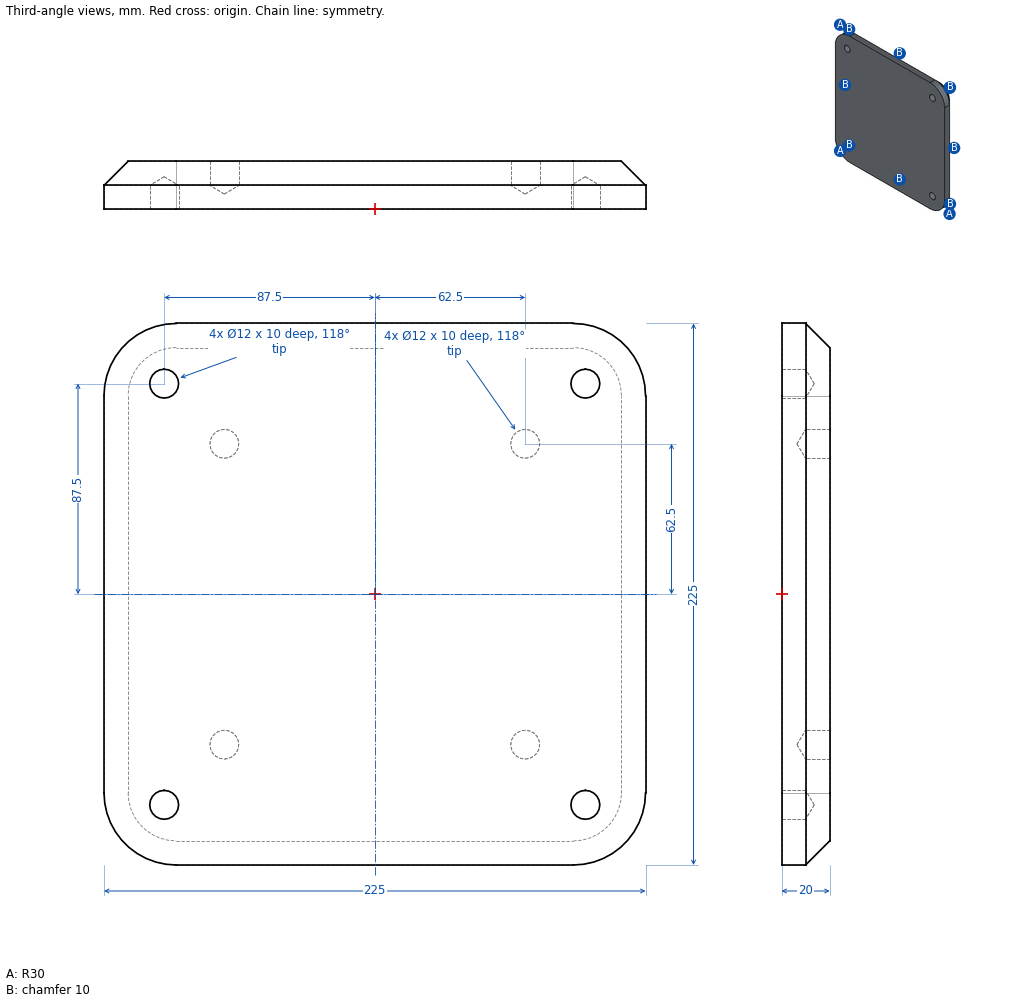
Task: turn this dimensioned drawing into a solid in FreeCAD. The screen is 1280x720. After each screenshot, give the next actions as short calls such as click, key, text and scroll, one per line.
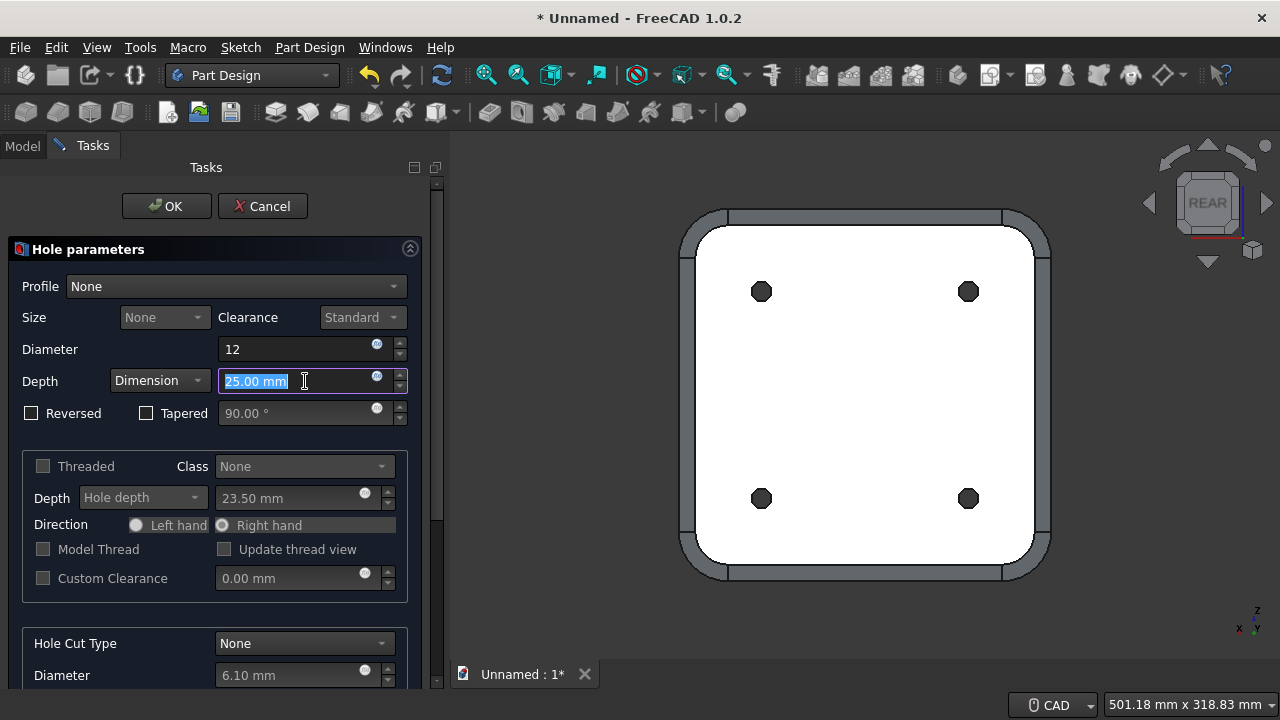
text(10)
key(Tab)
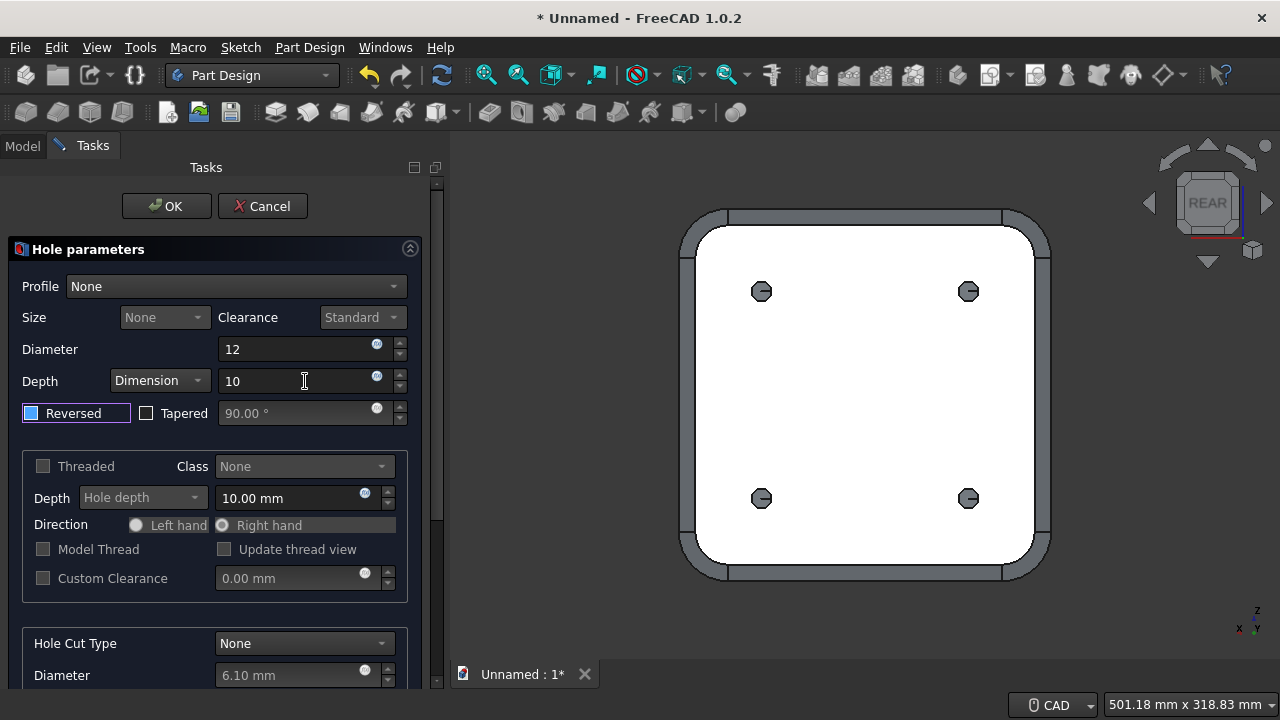
click(167, 206)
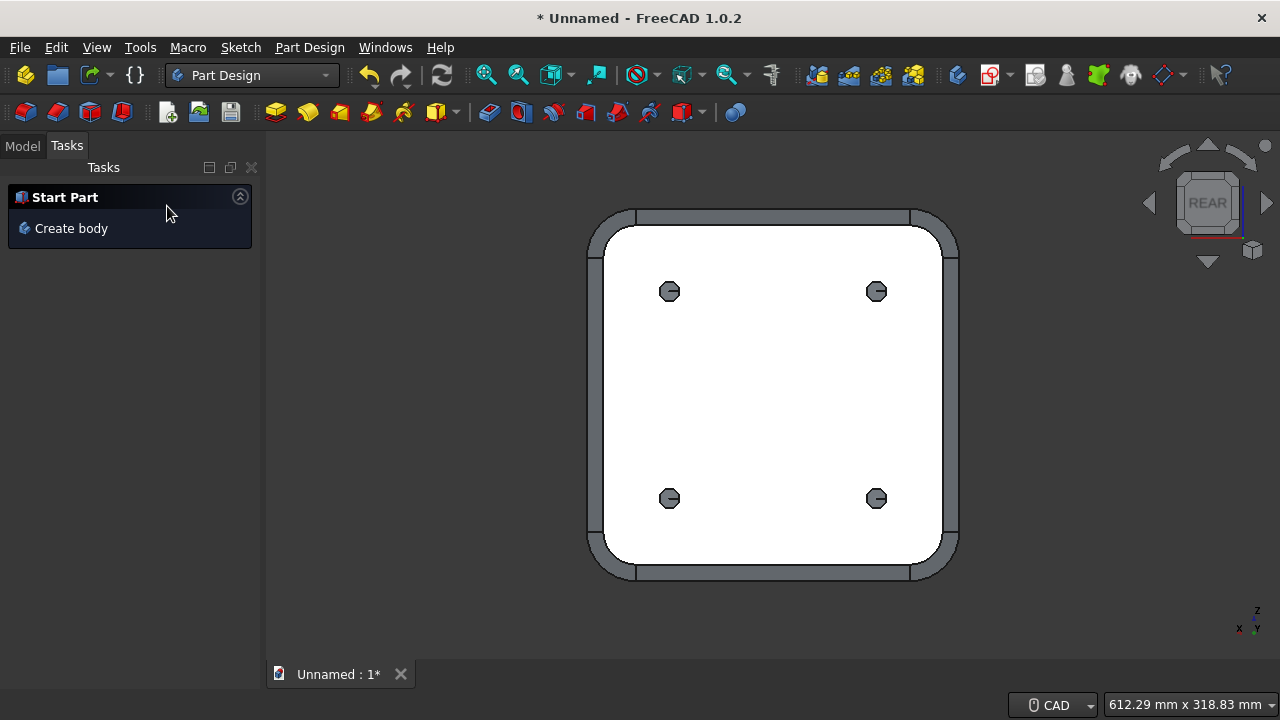
key(0)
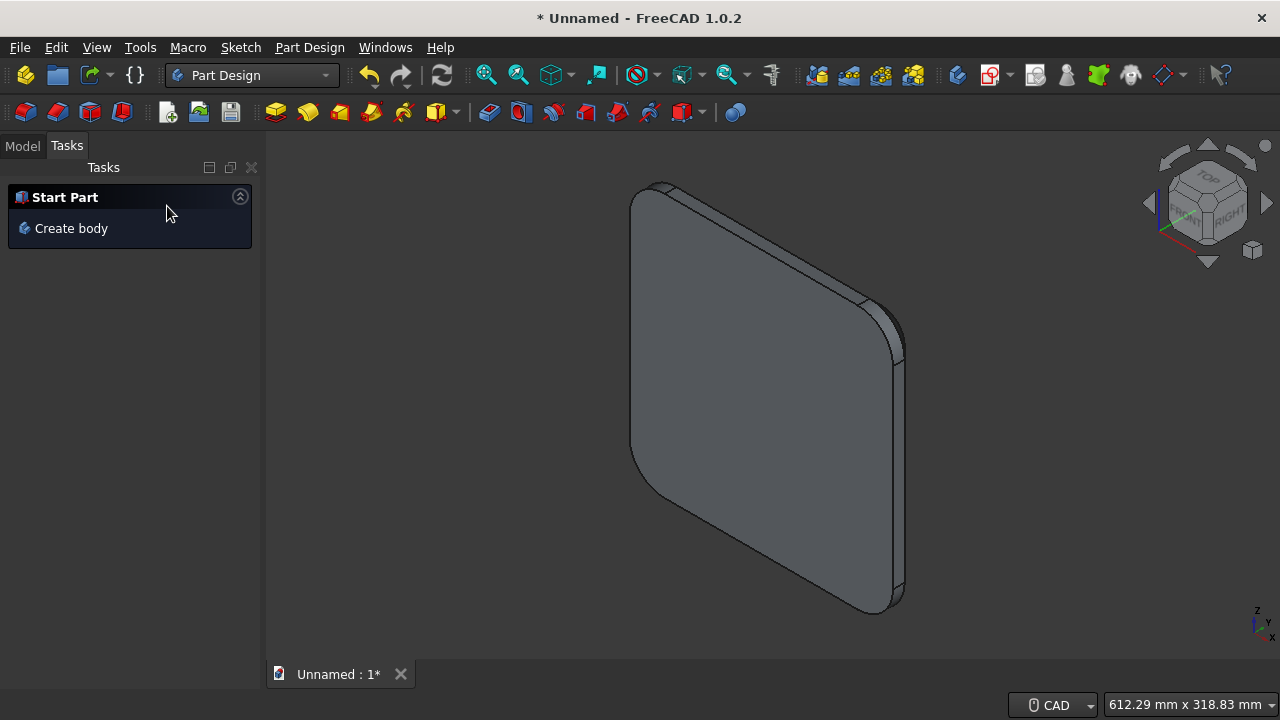
click(761, 401)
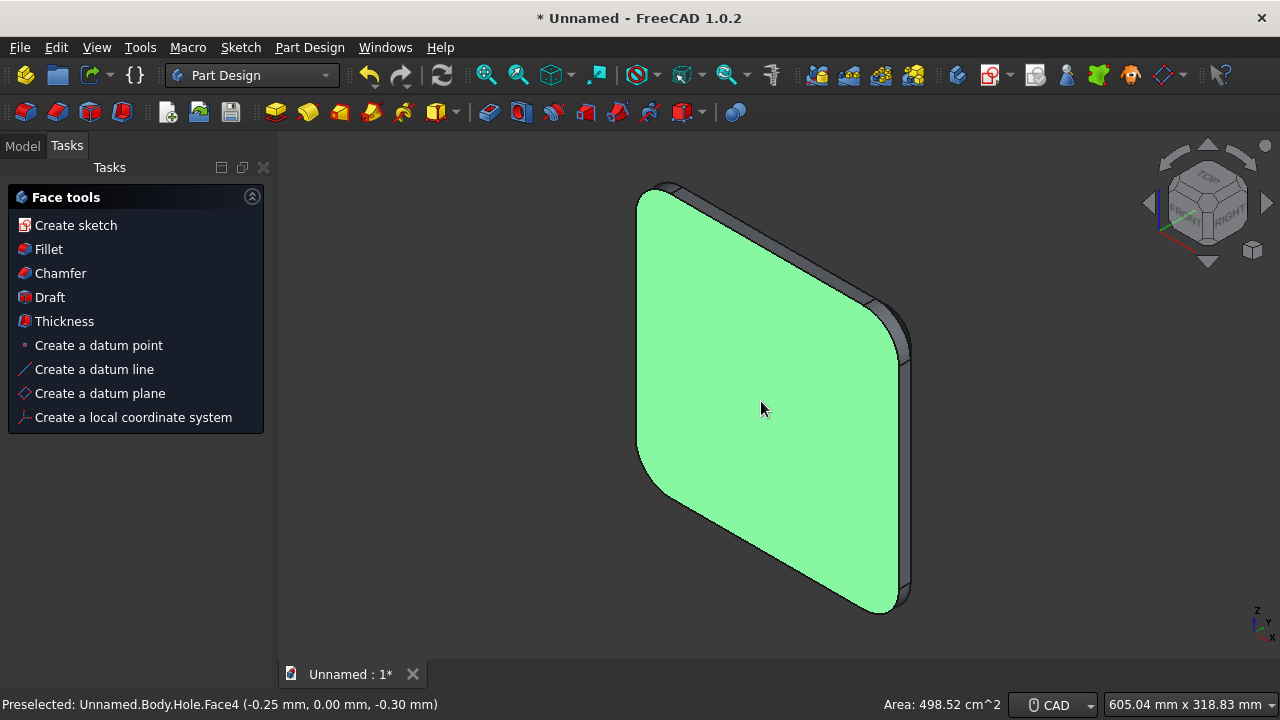
click(990, 76)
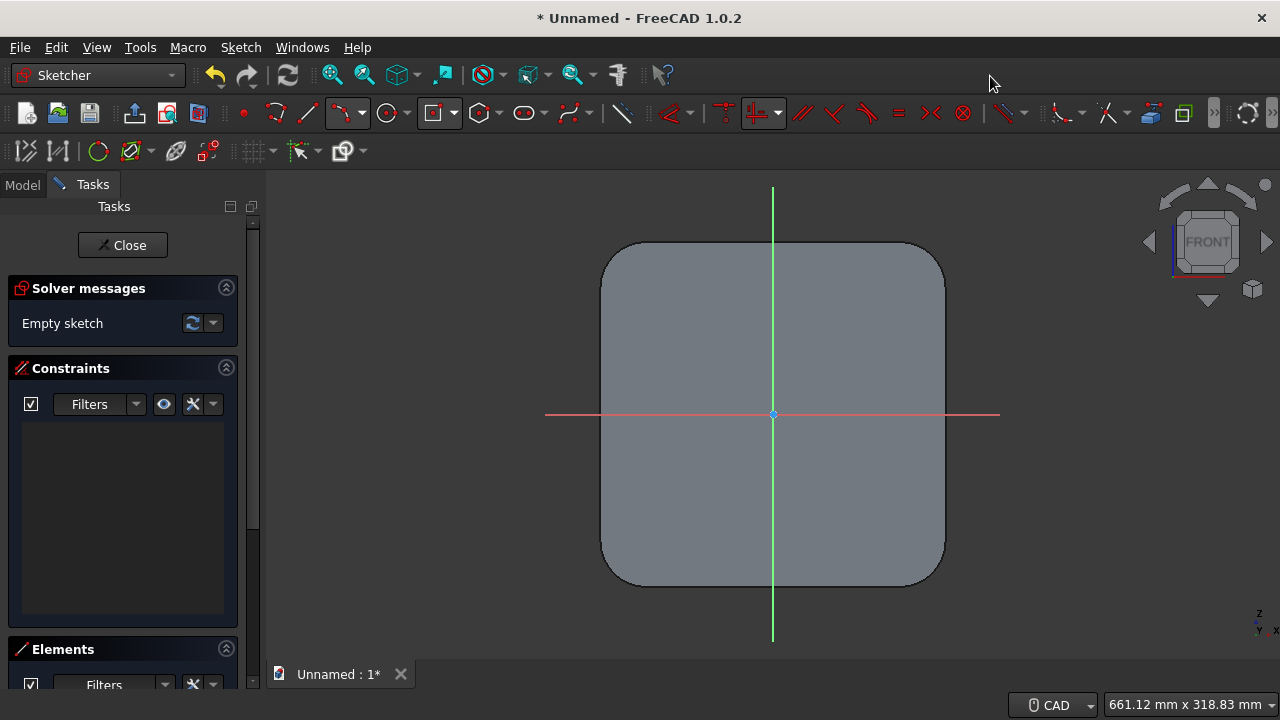
click(388, 114)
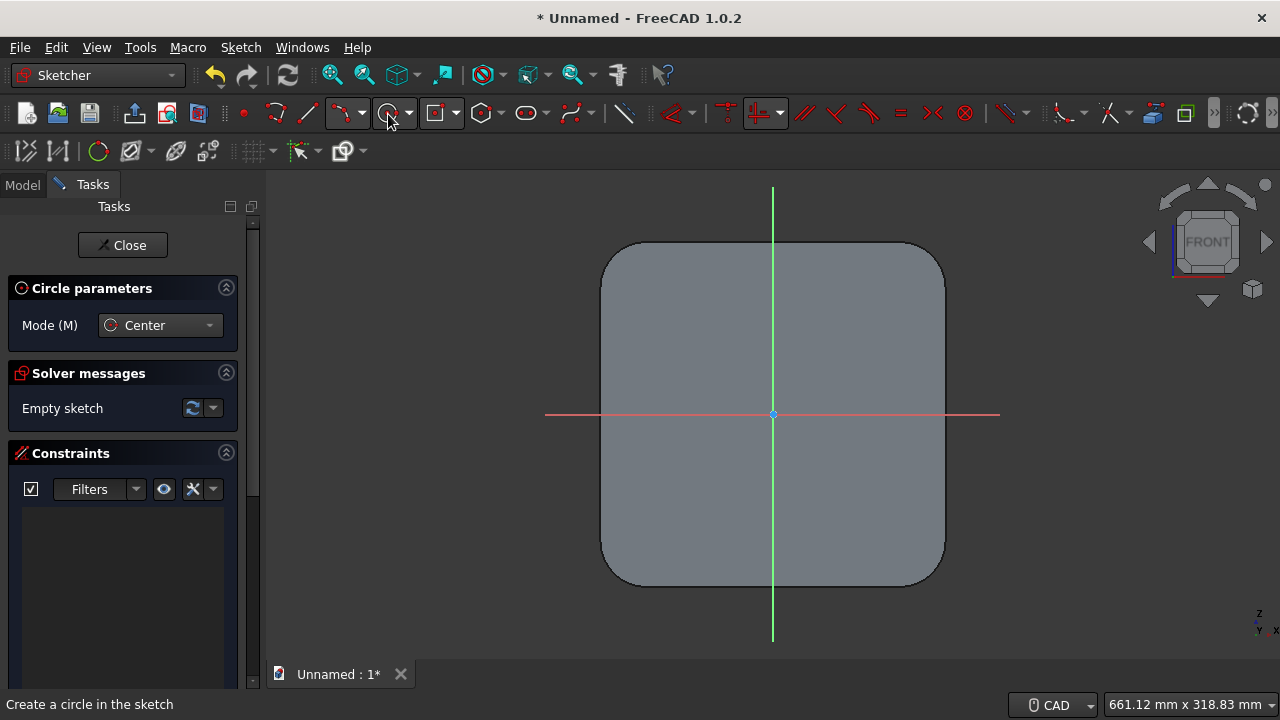
scroll(639, 280, up, 5)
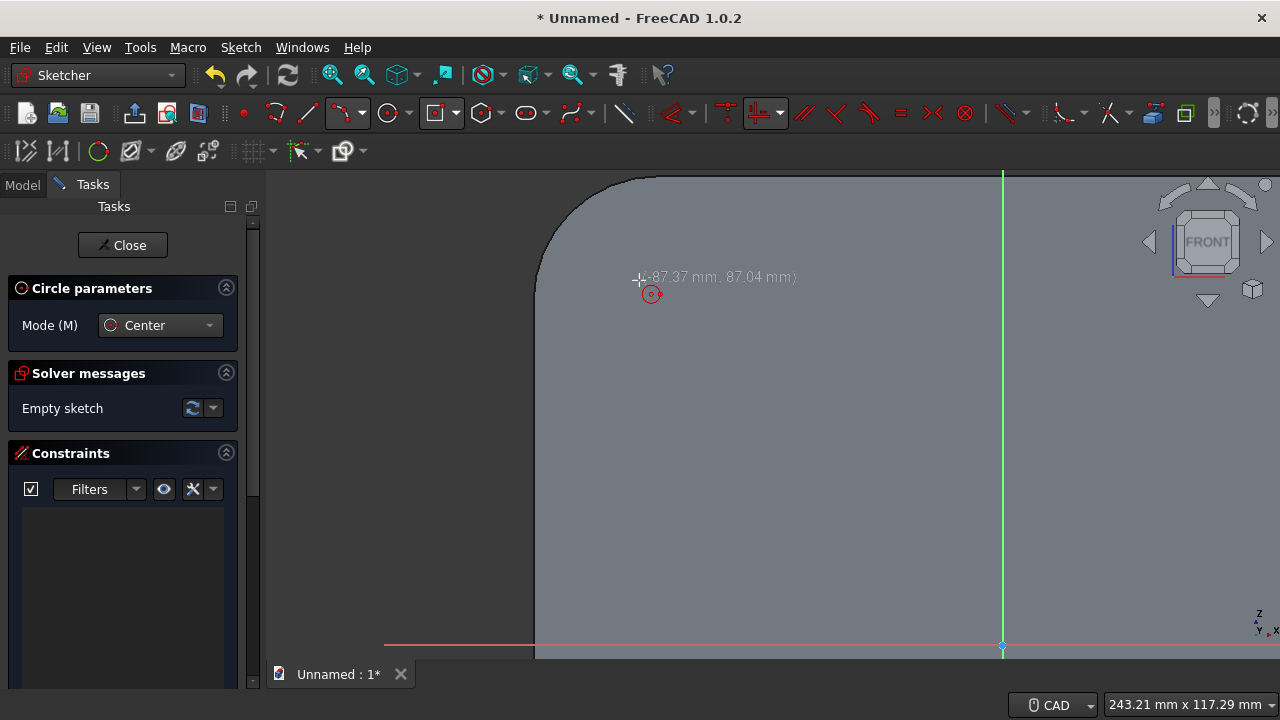
click(638, 280)
click(656, 263)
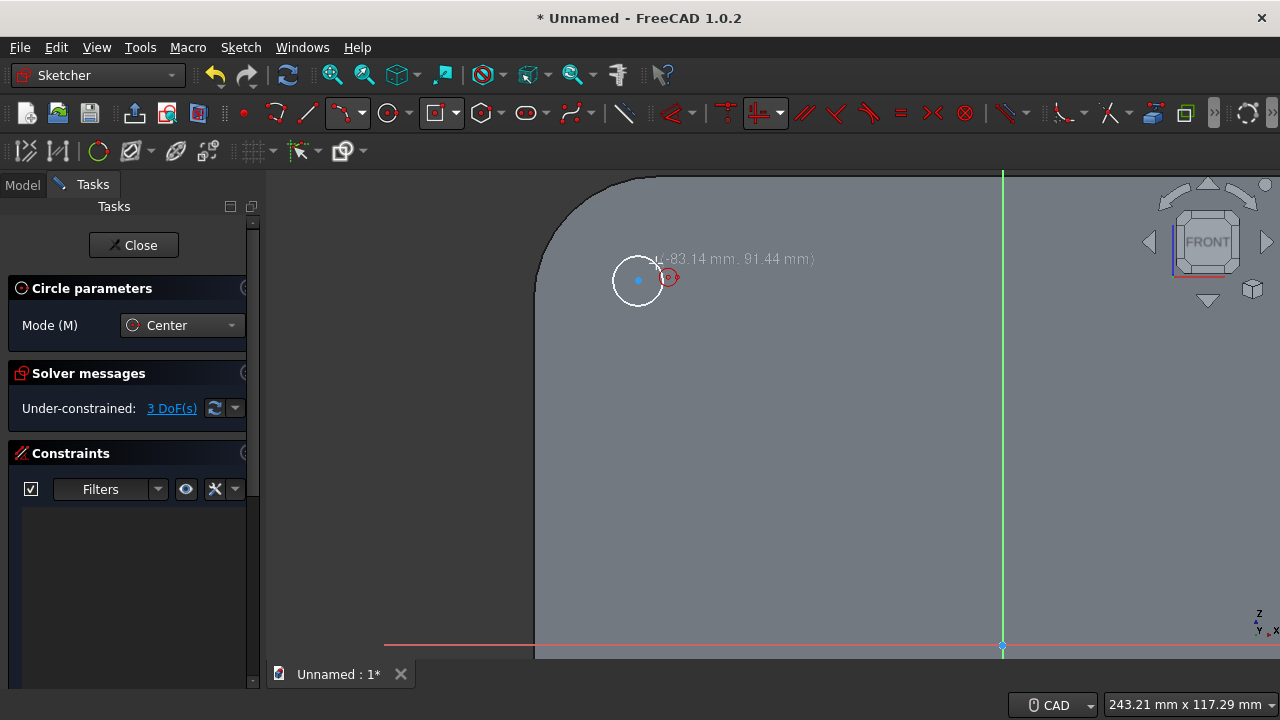
scroll(531, 280, down, 5)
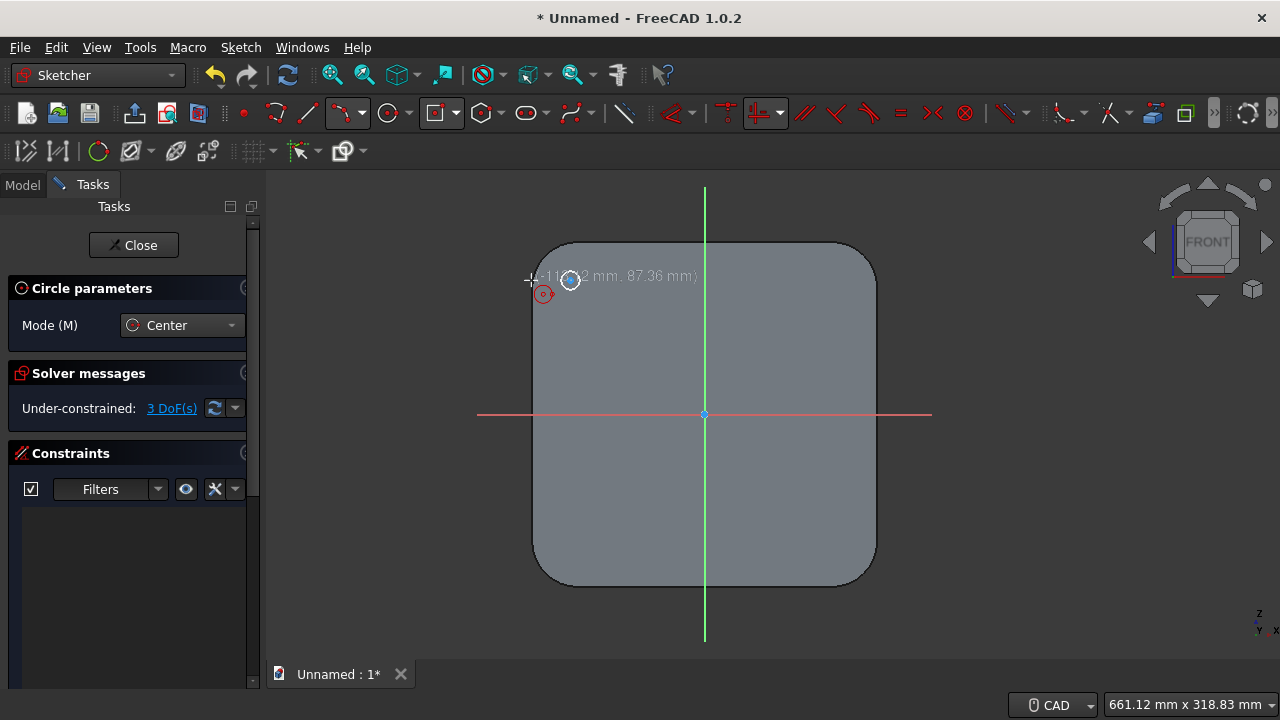
scroll(839, 280, up, 5)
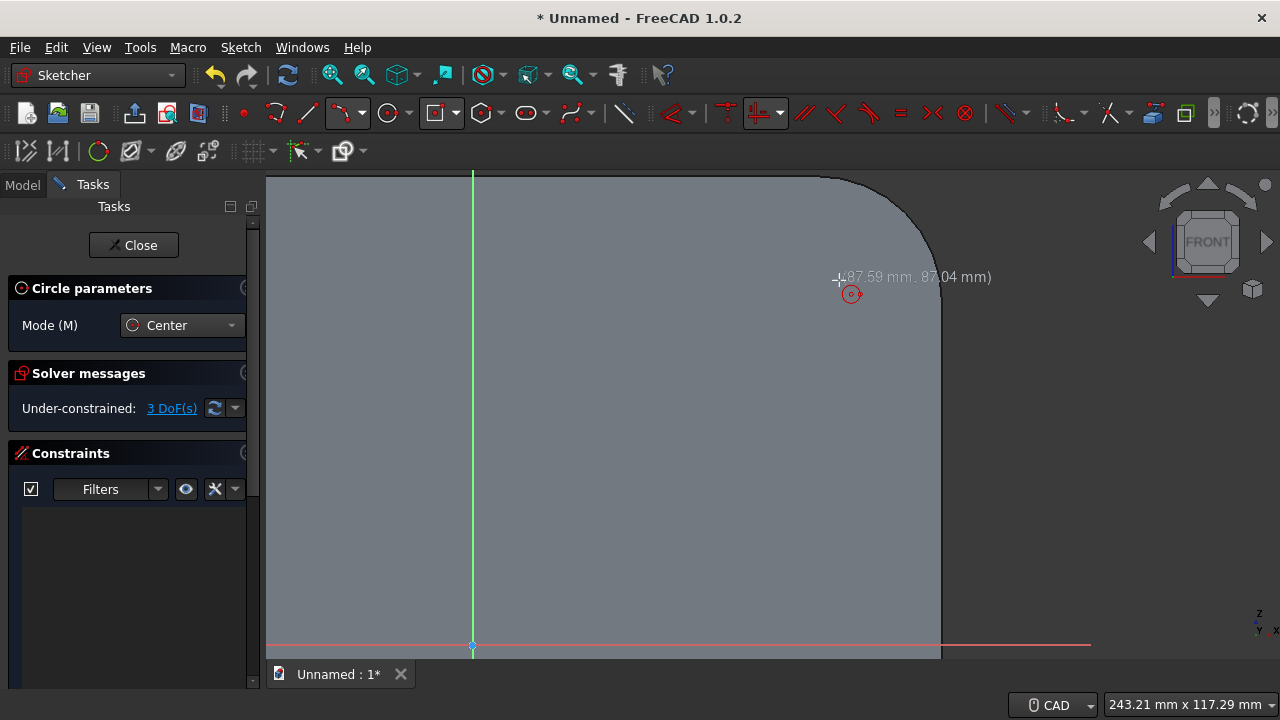
click(838, 280)
click(855, 263)